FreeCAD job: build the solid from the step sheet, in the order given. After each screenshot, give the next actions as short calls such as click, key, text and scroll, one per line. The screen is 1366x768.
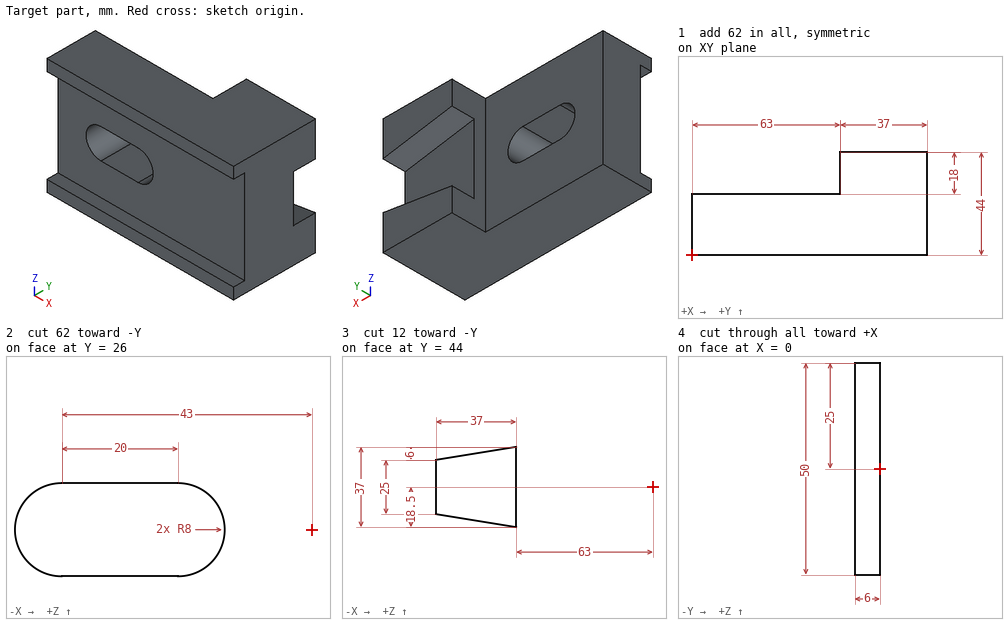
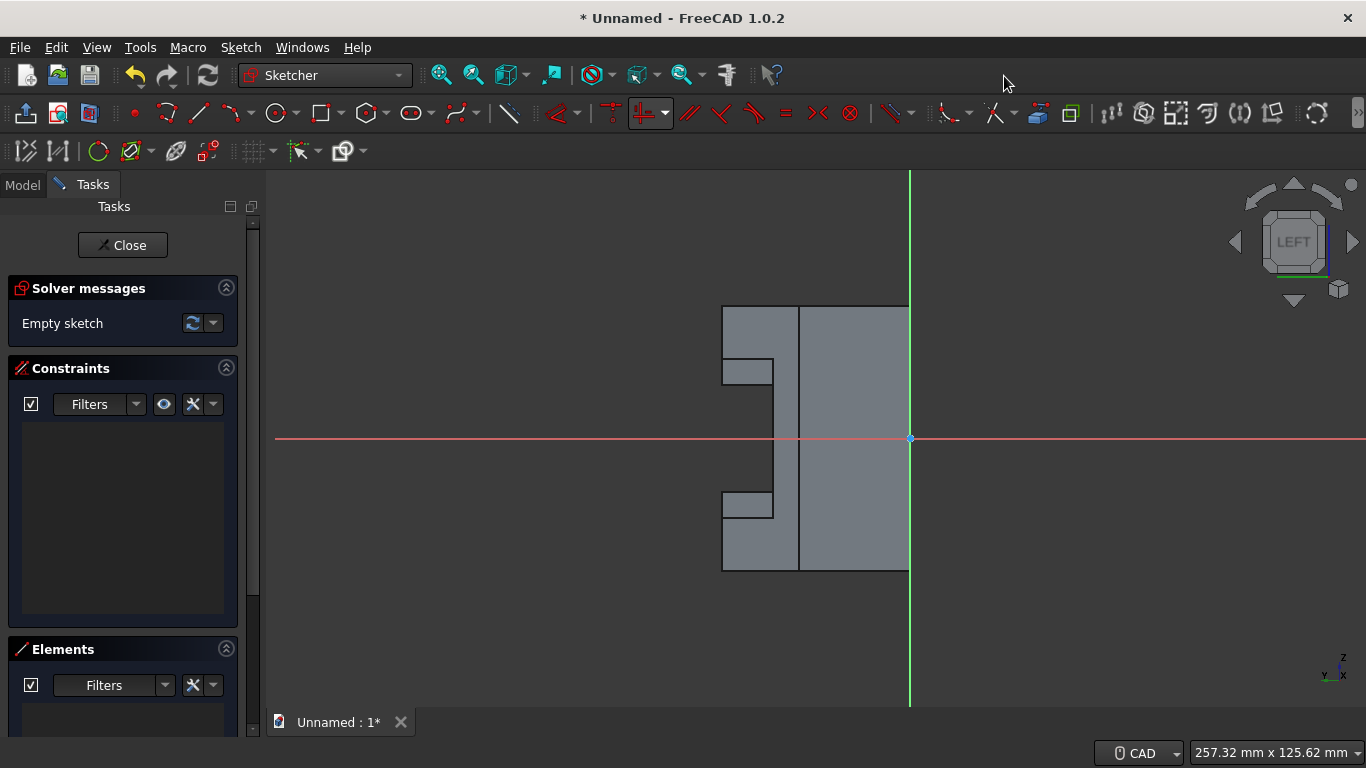
scroll(1201, 439, up, 2)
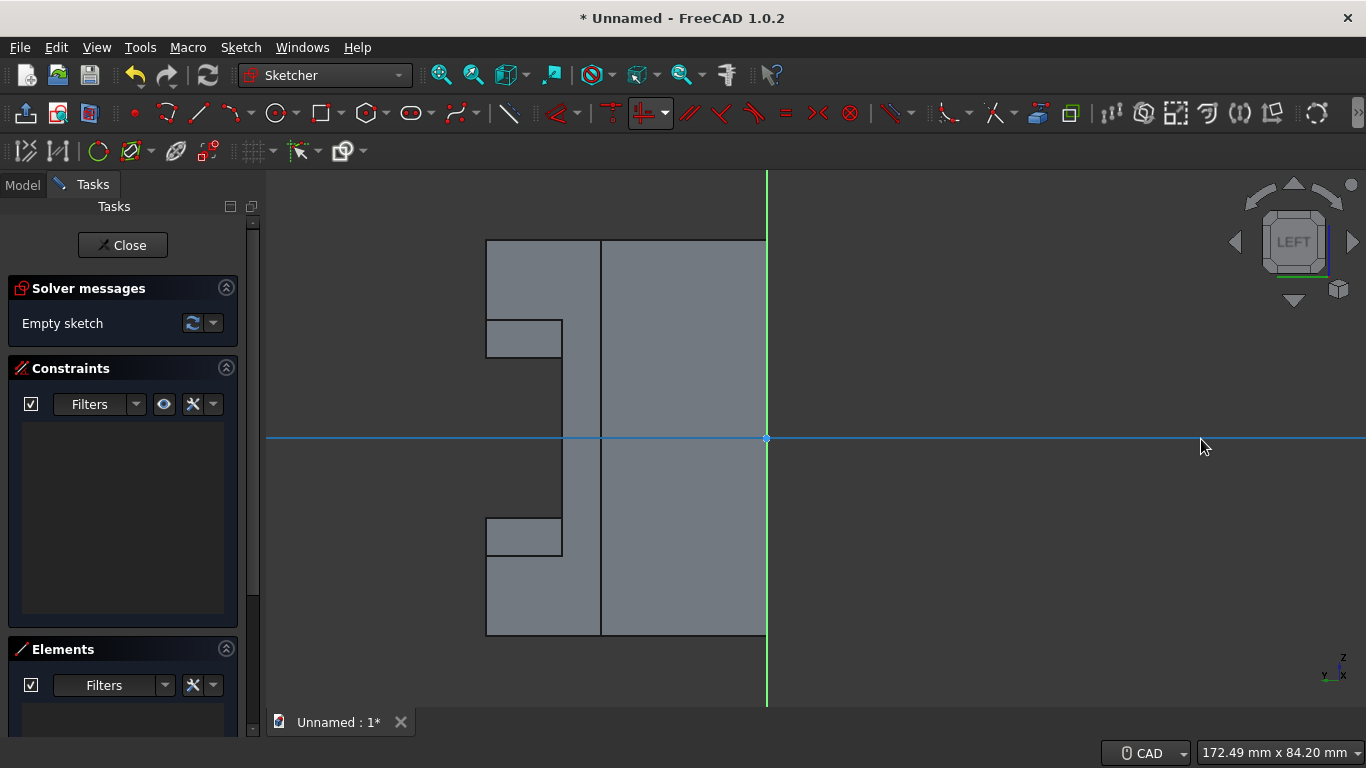
click(322, 114)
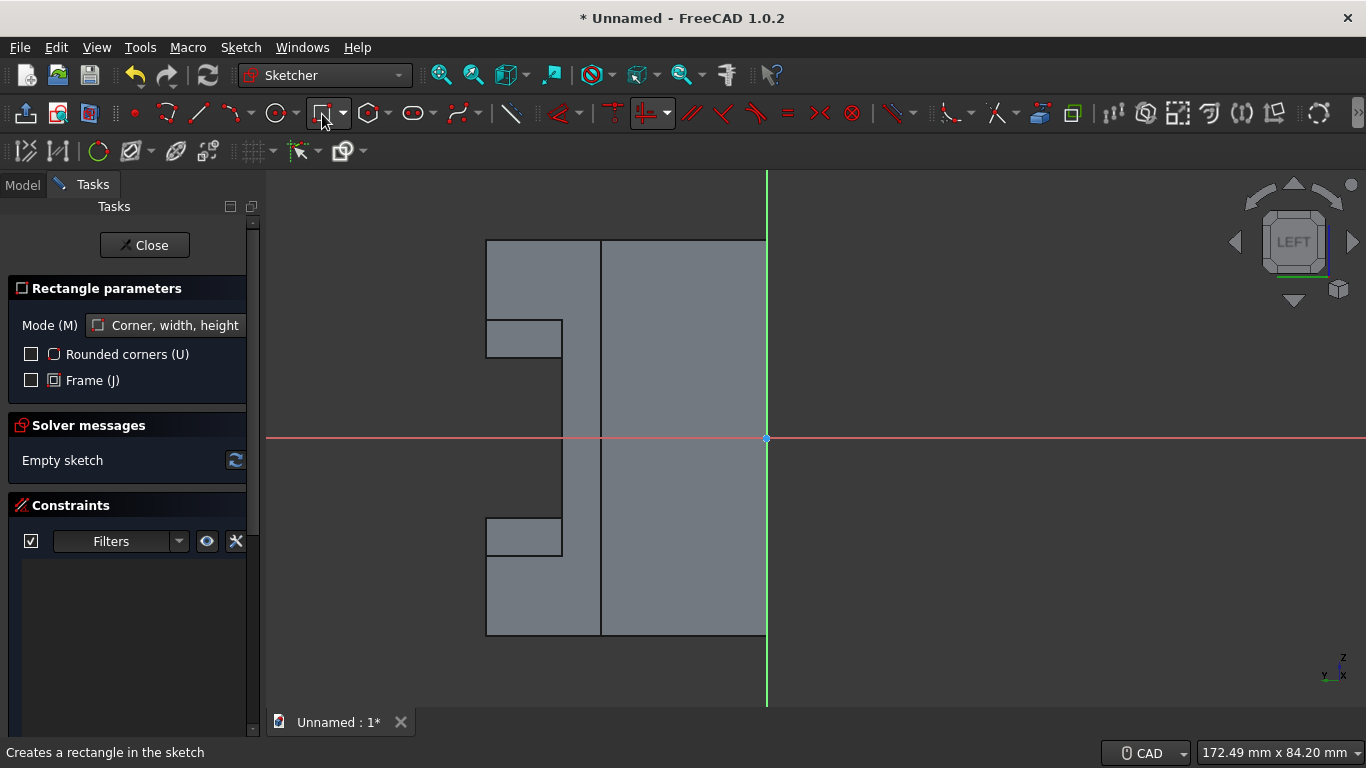
click(728, 279)
click(767, 597)
key(Escape)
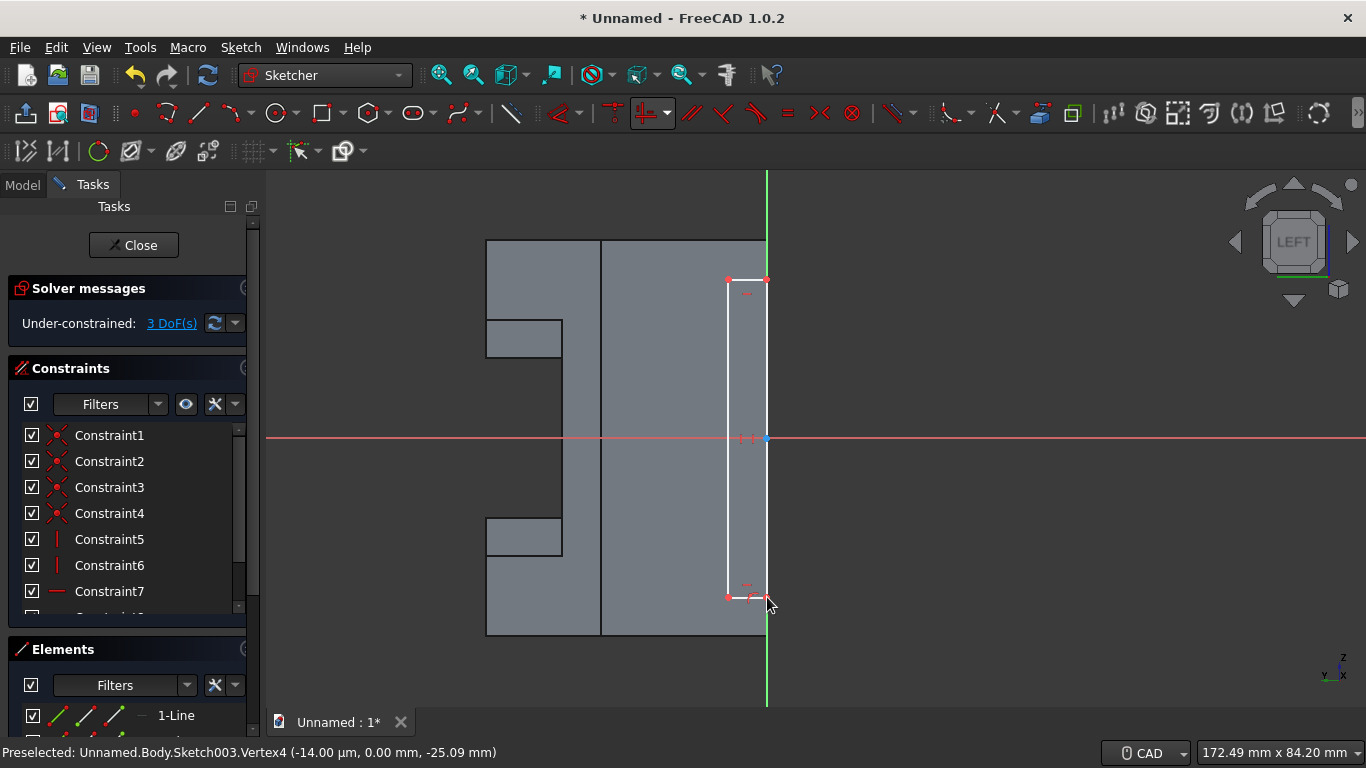
click(558, 114)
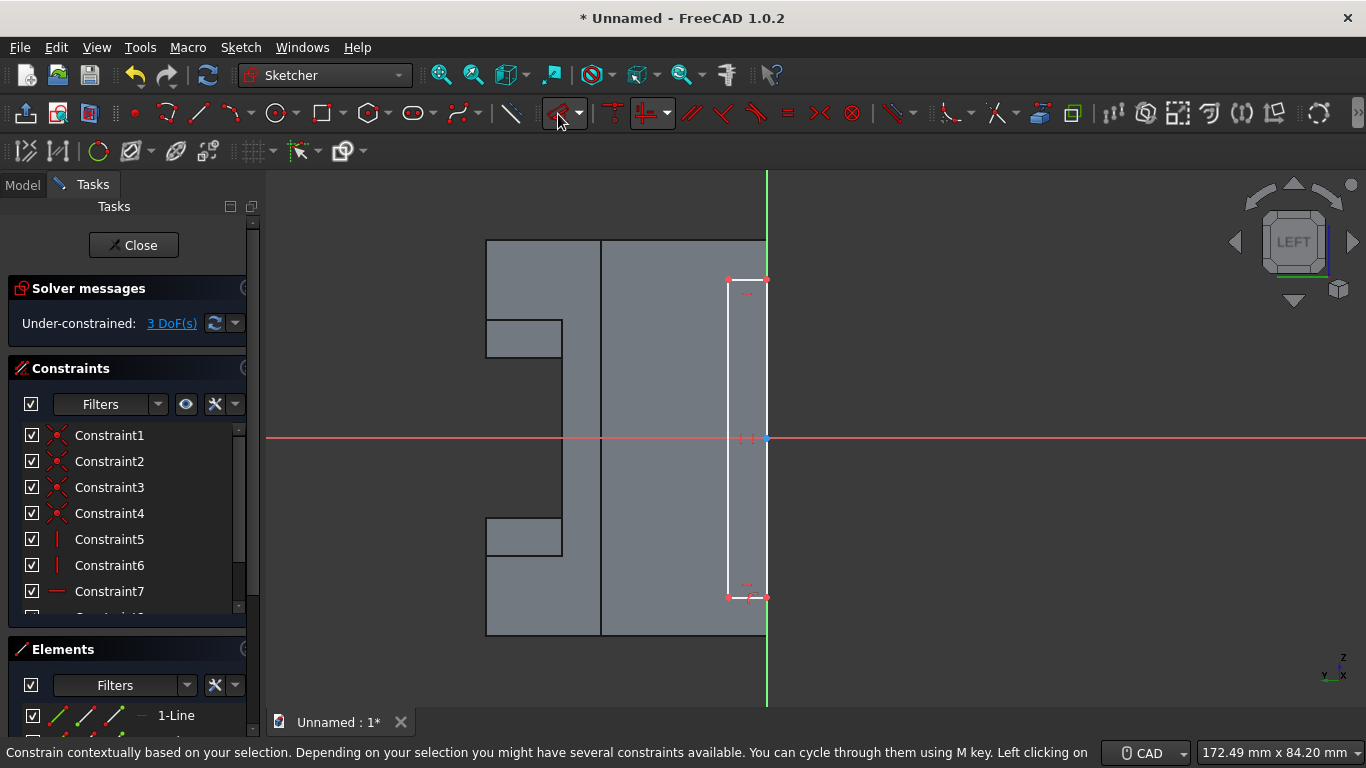
click(740, 598)
click(747, 632)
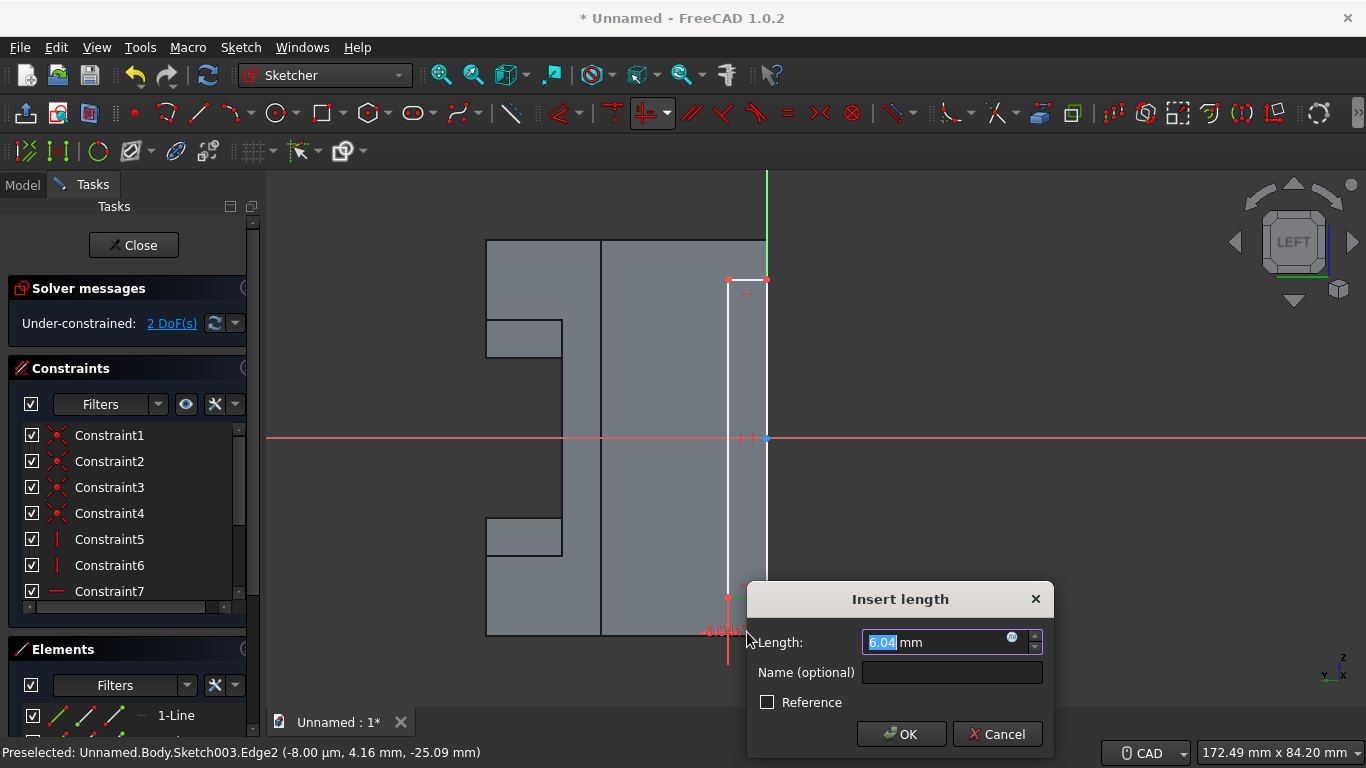
text(6)
key(Return)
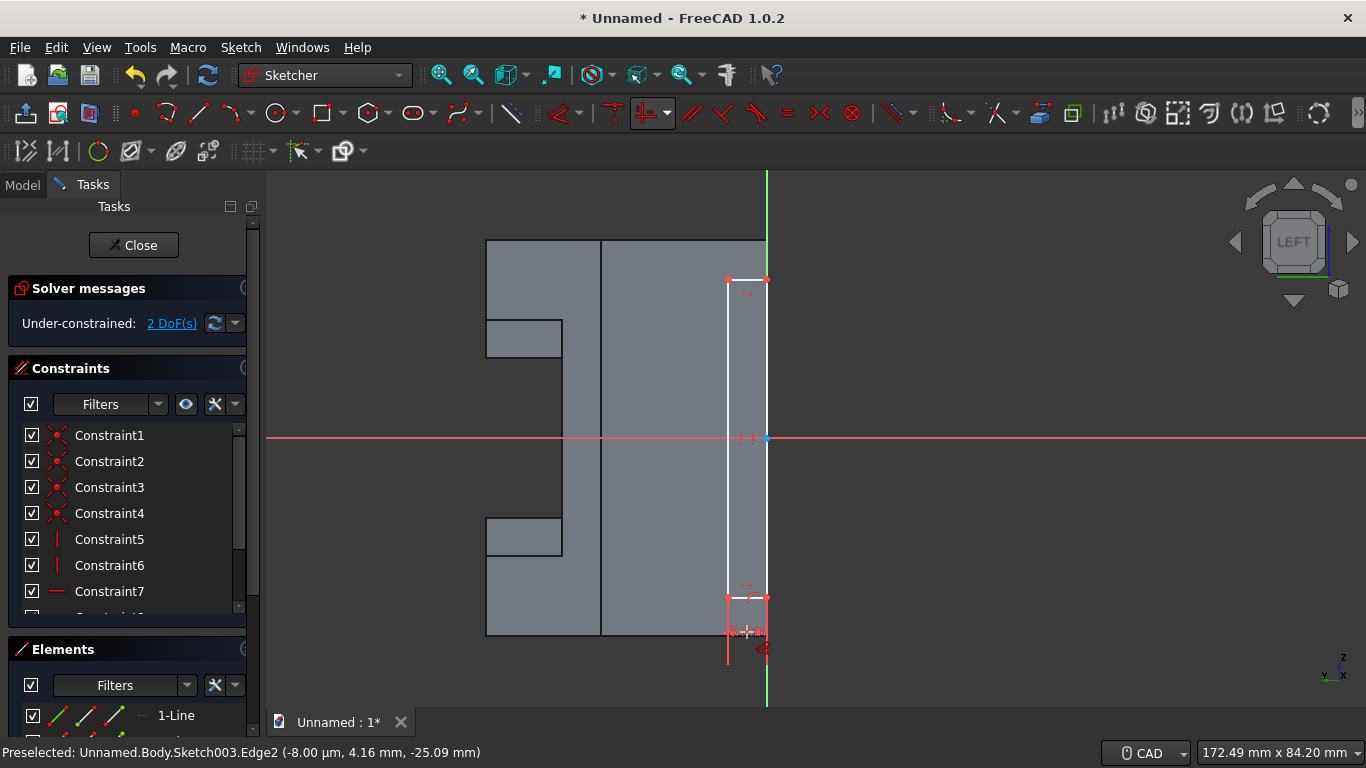
click(728, 375)
click(694, 366)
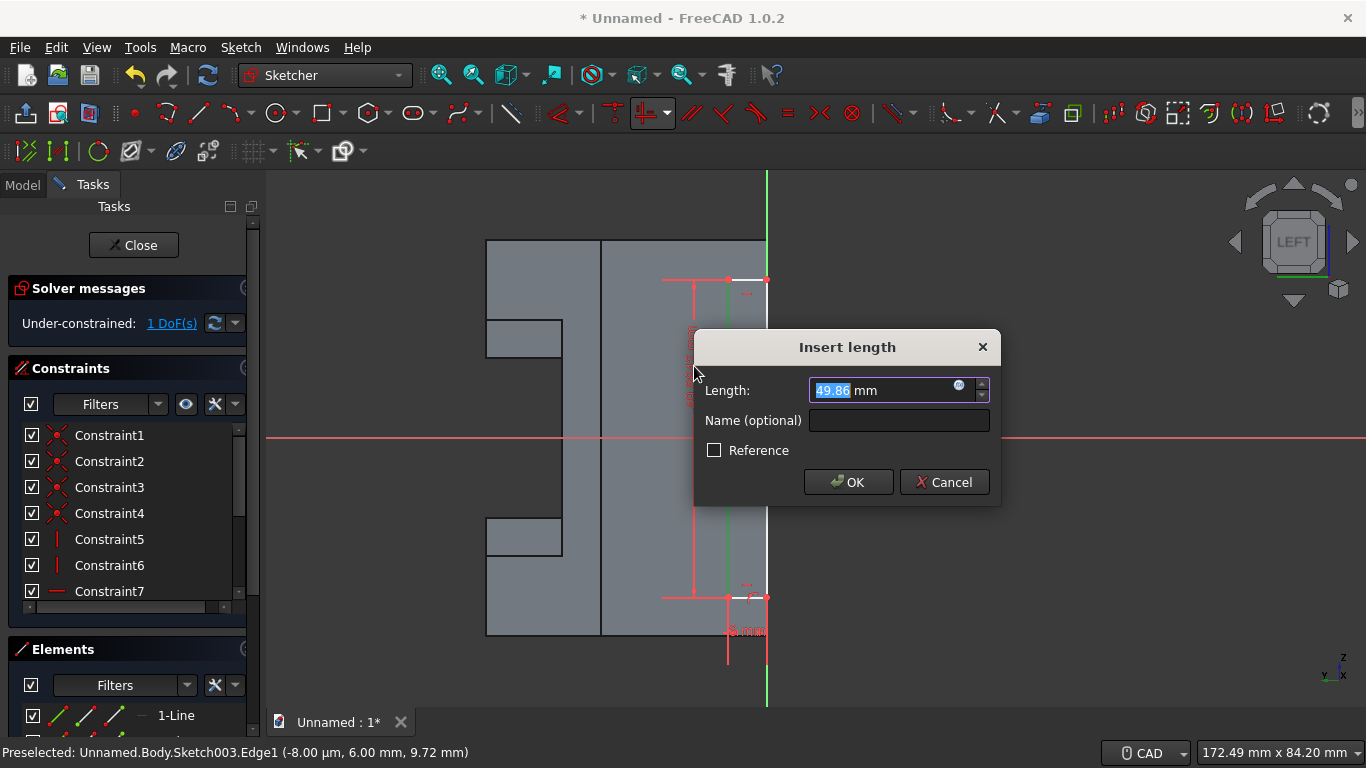
text(50)
key(Return)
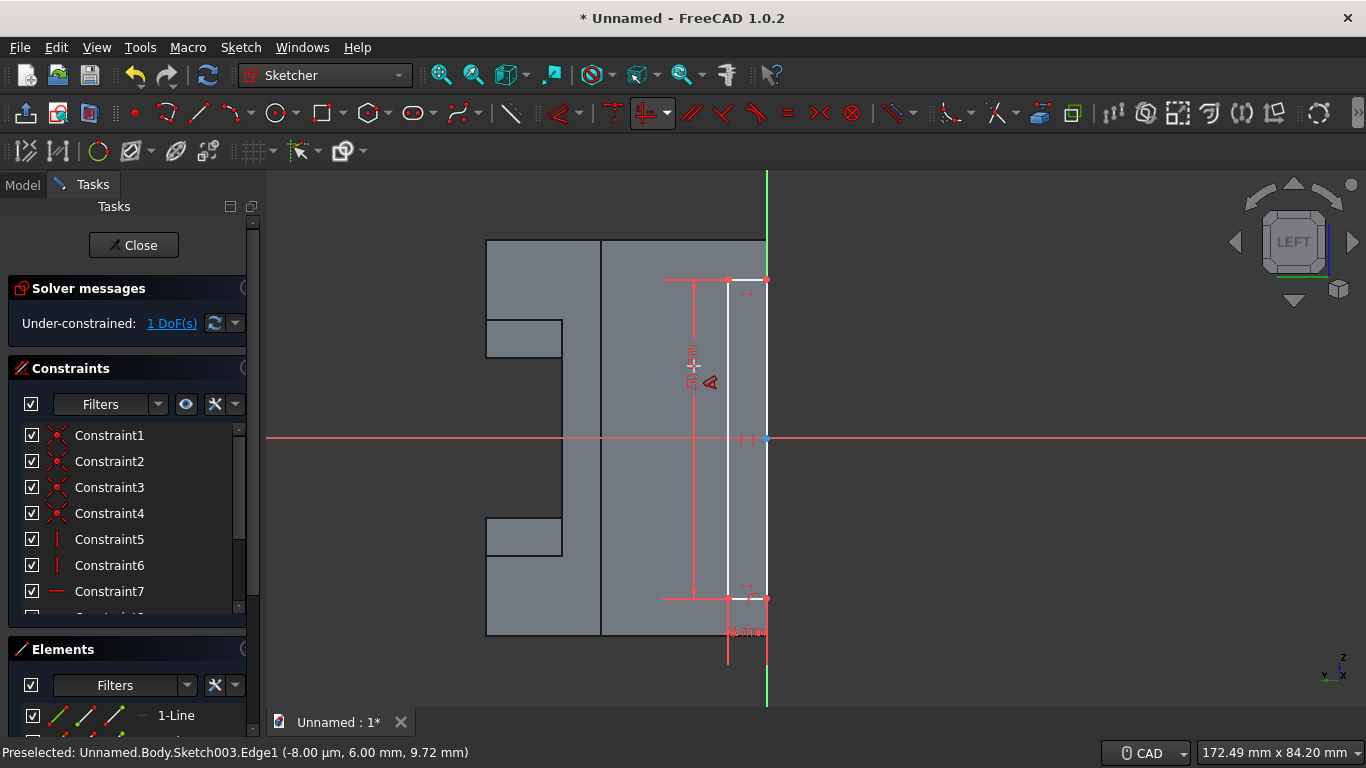
click(728, 280)
click(801, 359)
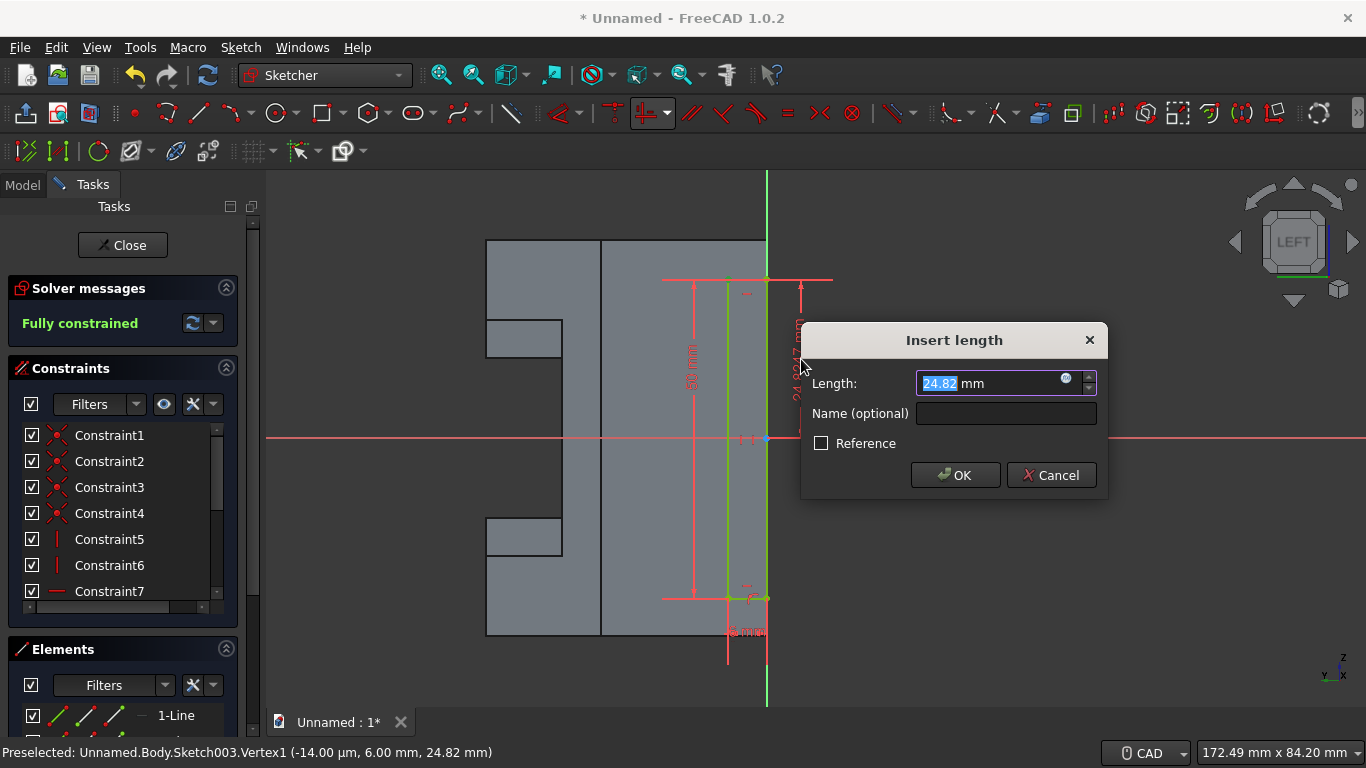
text(25)
key(Return)
key(Escape)